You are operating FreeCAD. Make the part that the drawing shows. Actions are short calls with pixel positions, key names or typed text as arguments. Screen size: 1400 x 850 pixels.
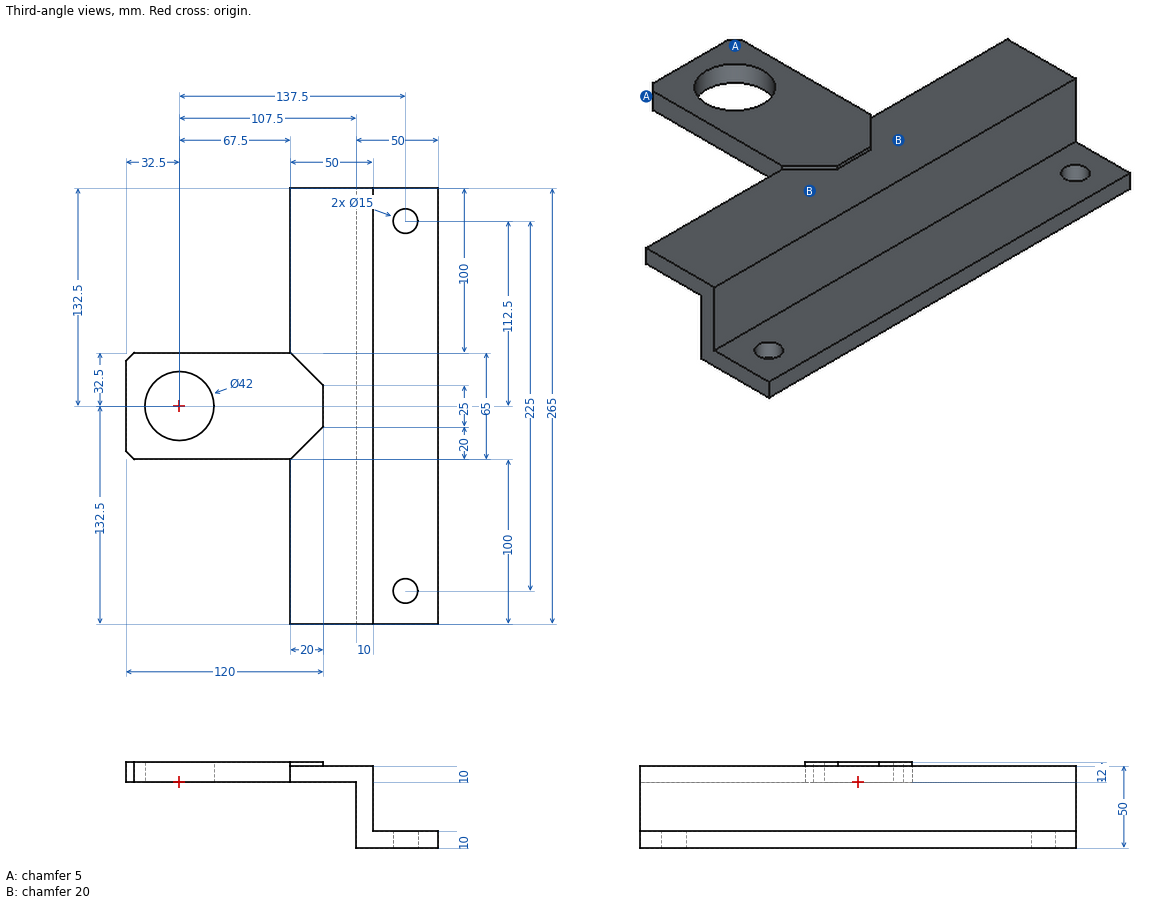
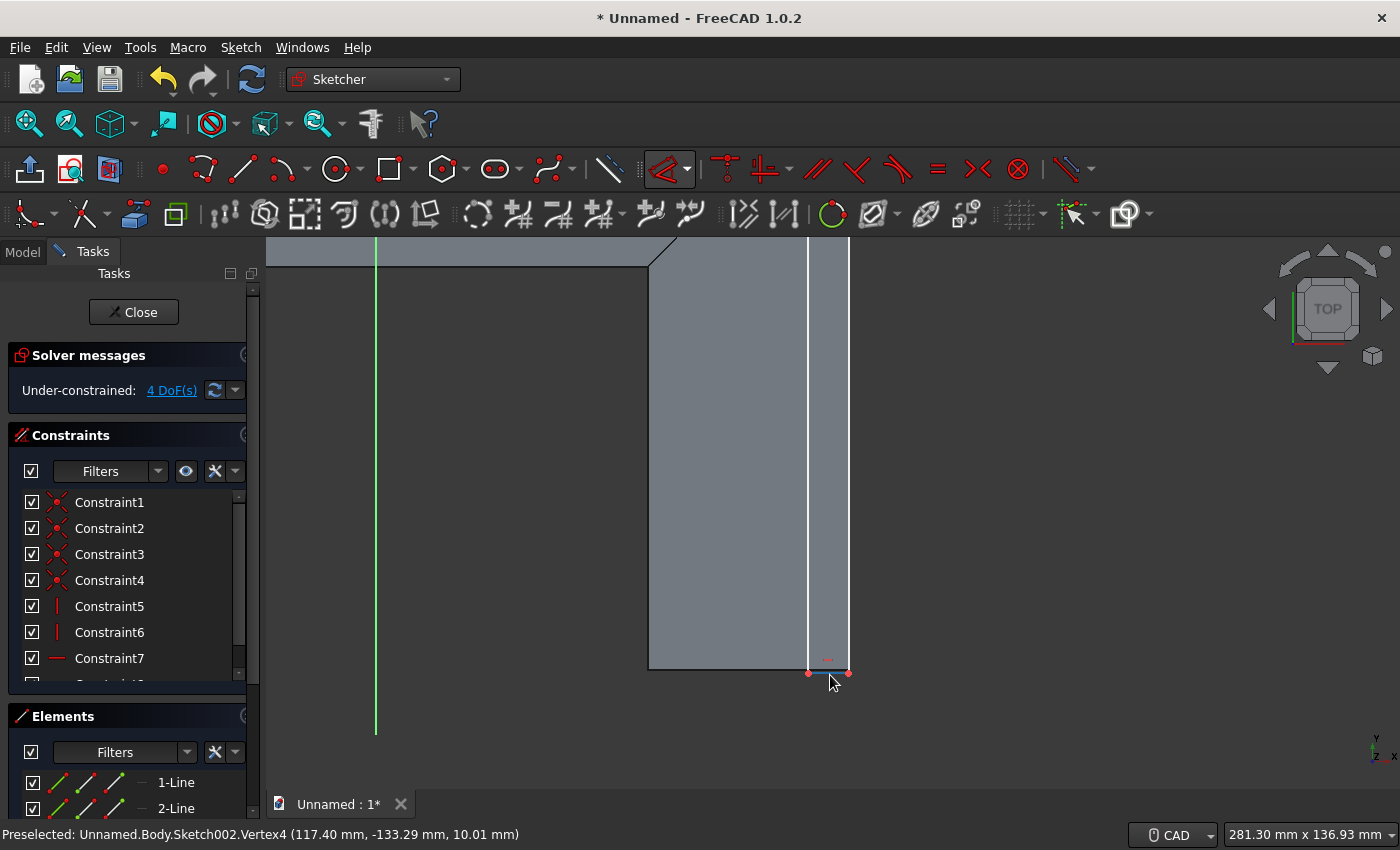
click(829, 673)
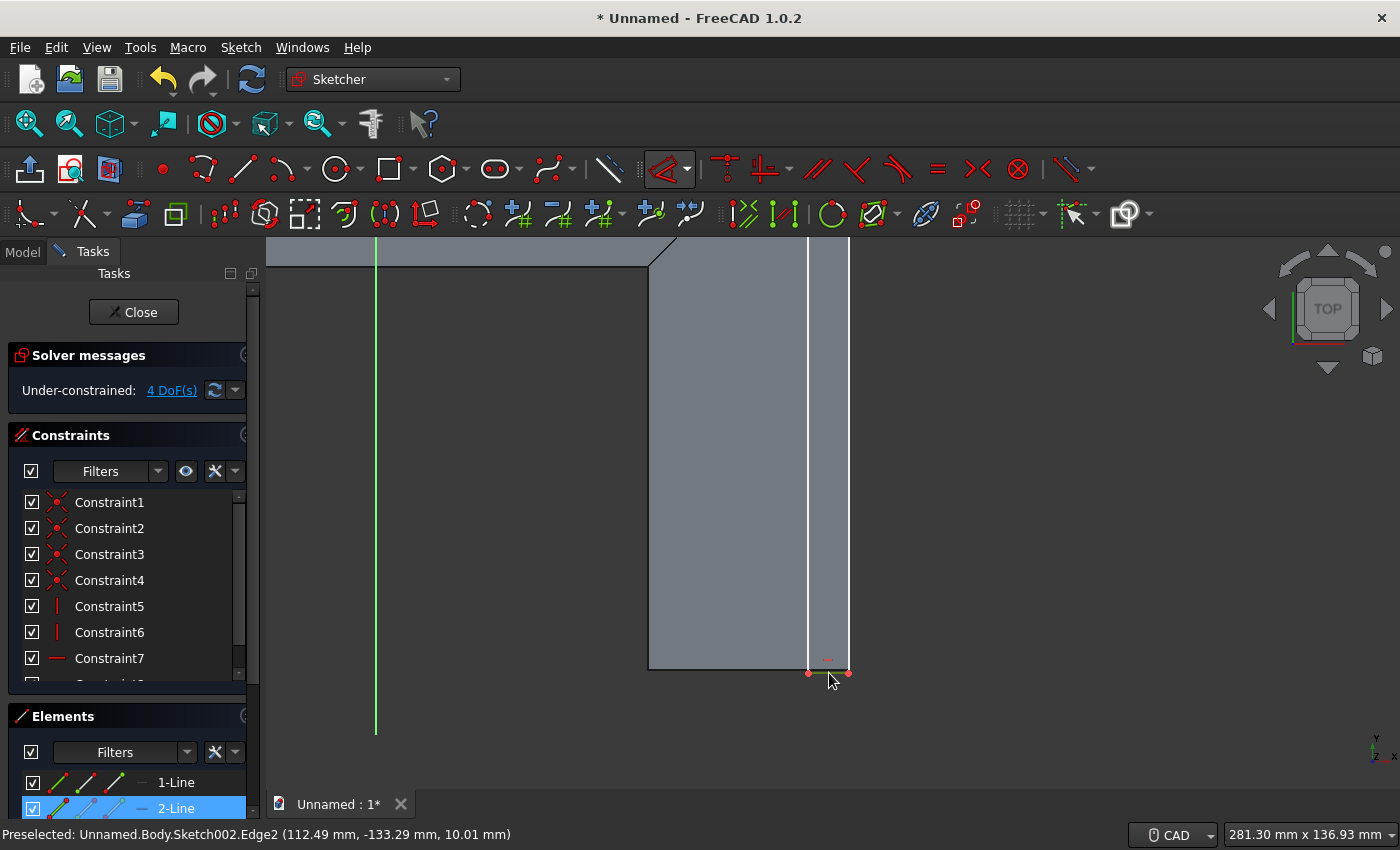
key(l)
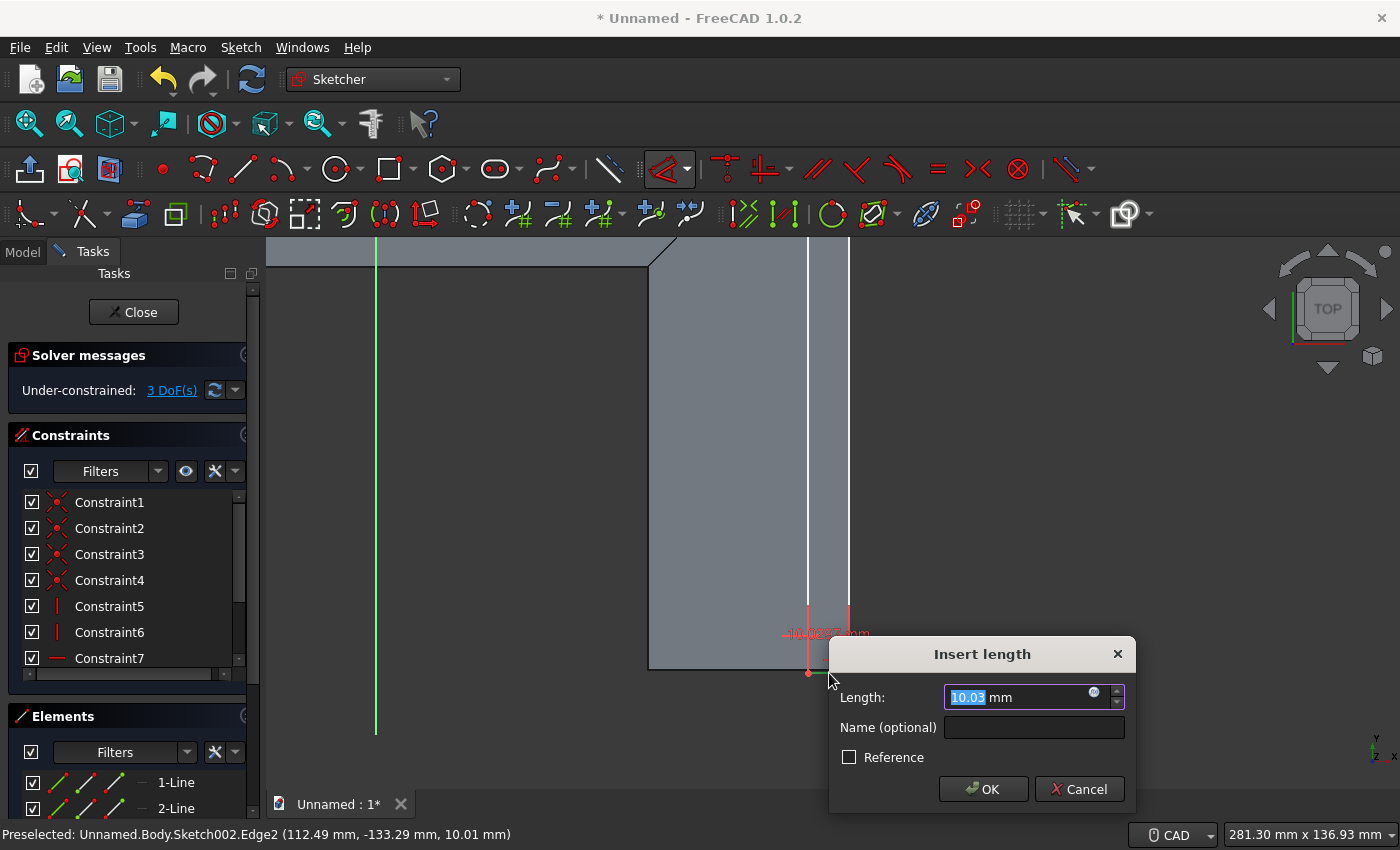
text(10)
key(Return)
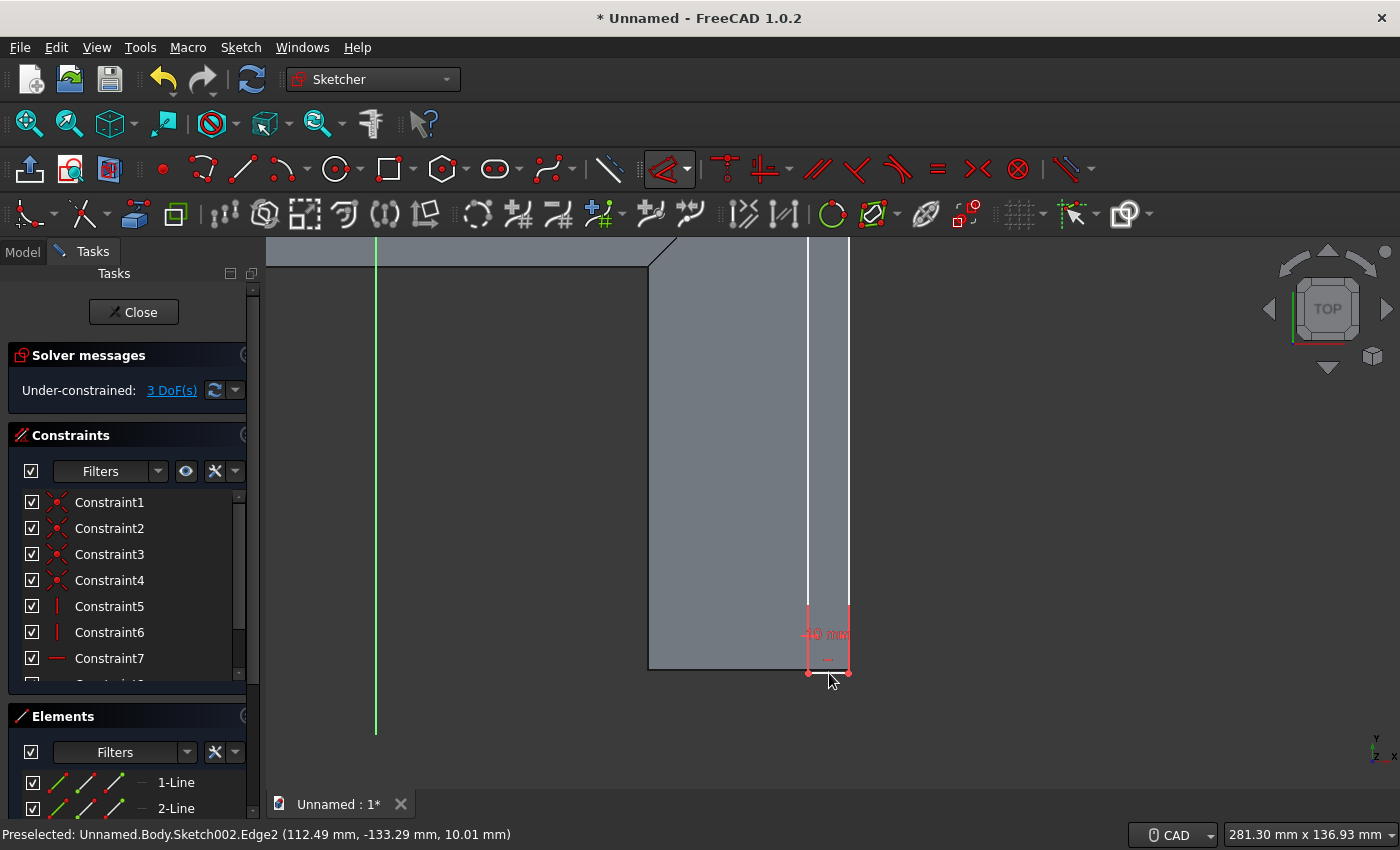
click(808, 352)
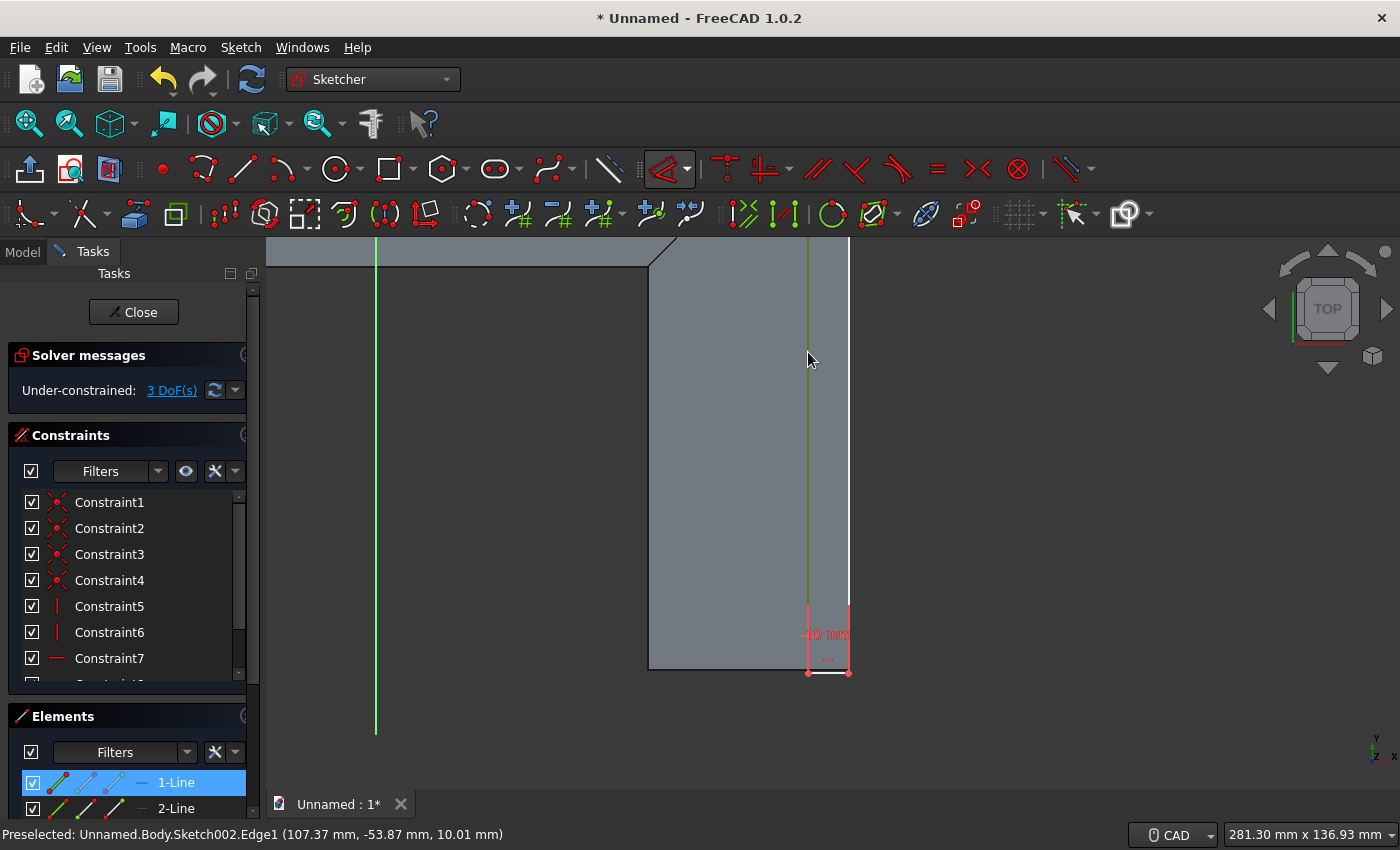
key(i)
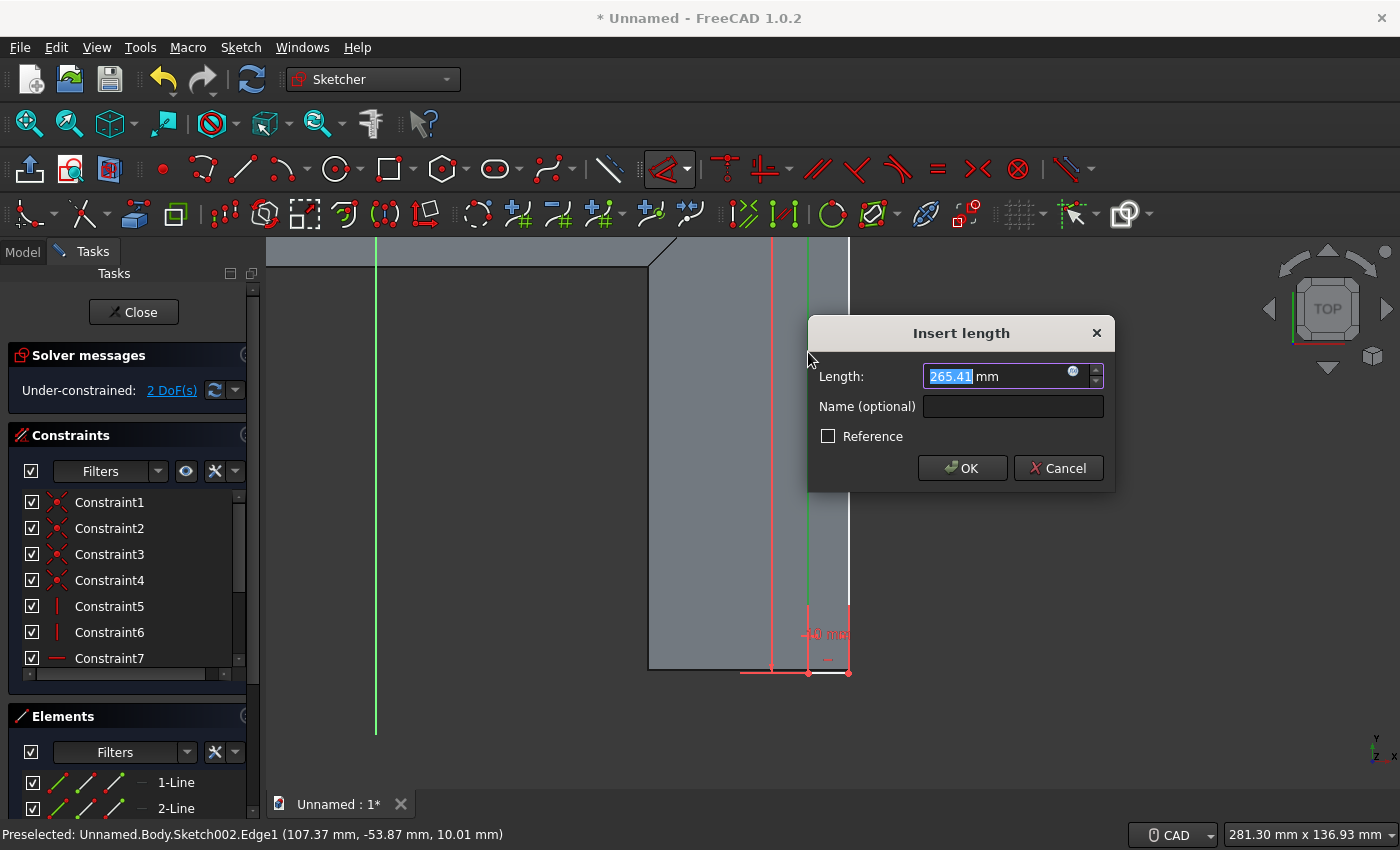
text(265)
key(Return)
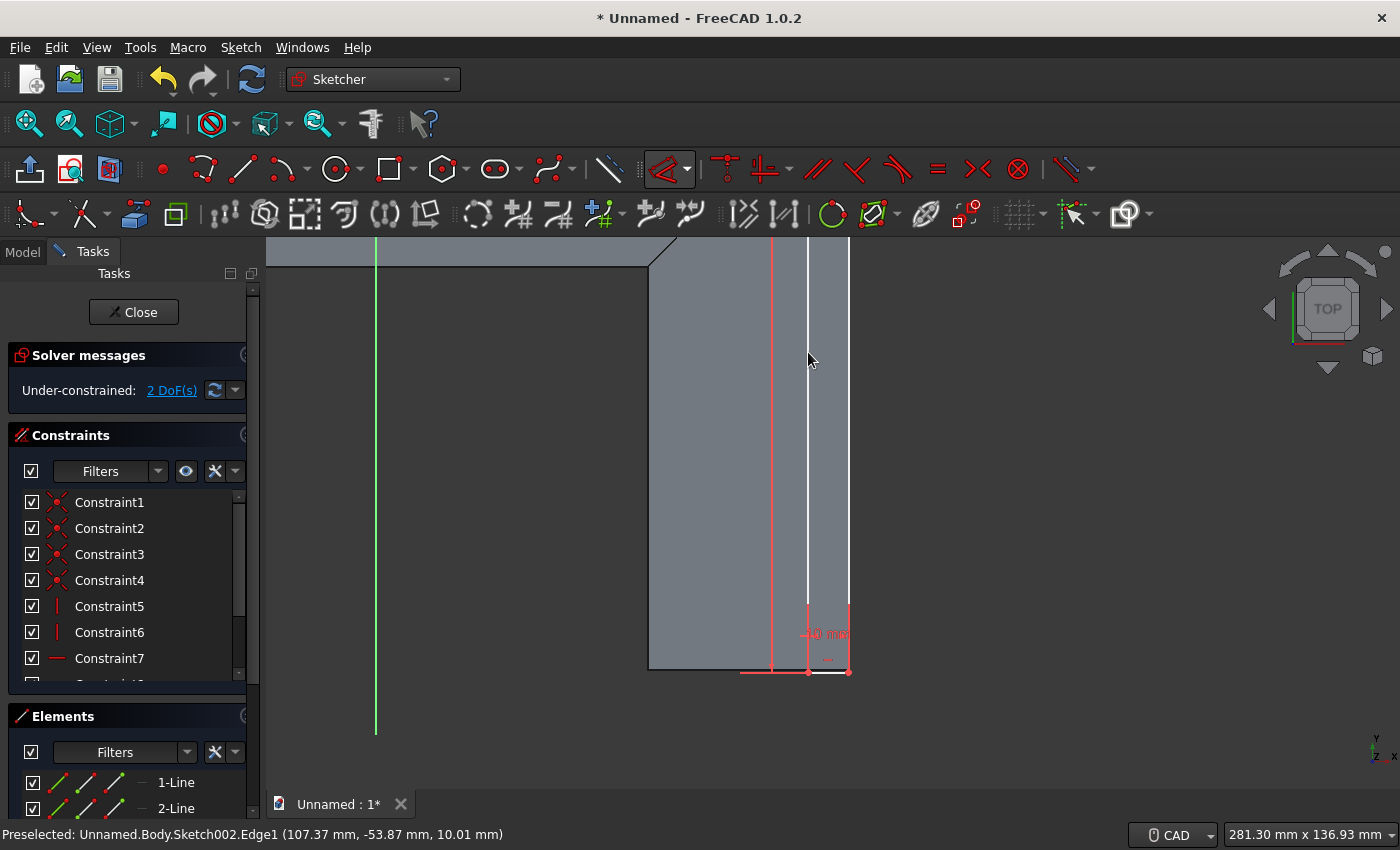
scroll(830, 676, down, 6)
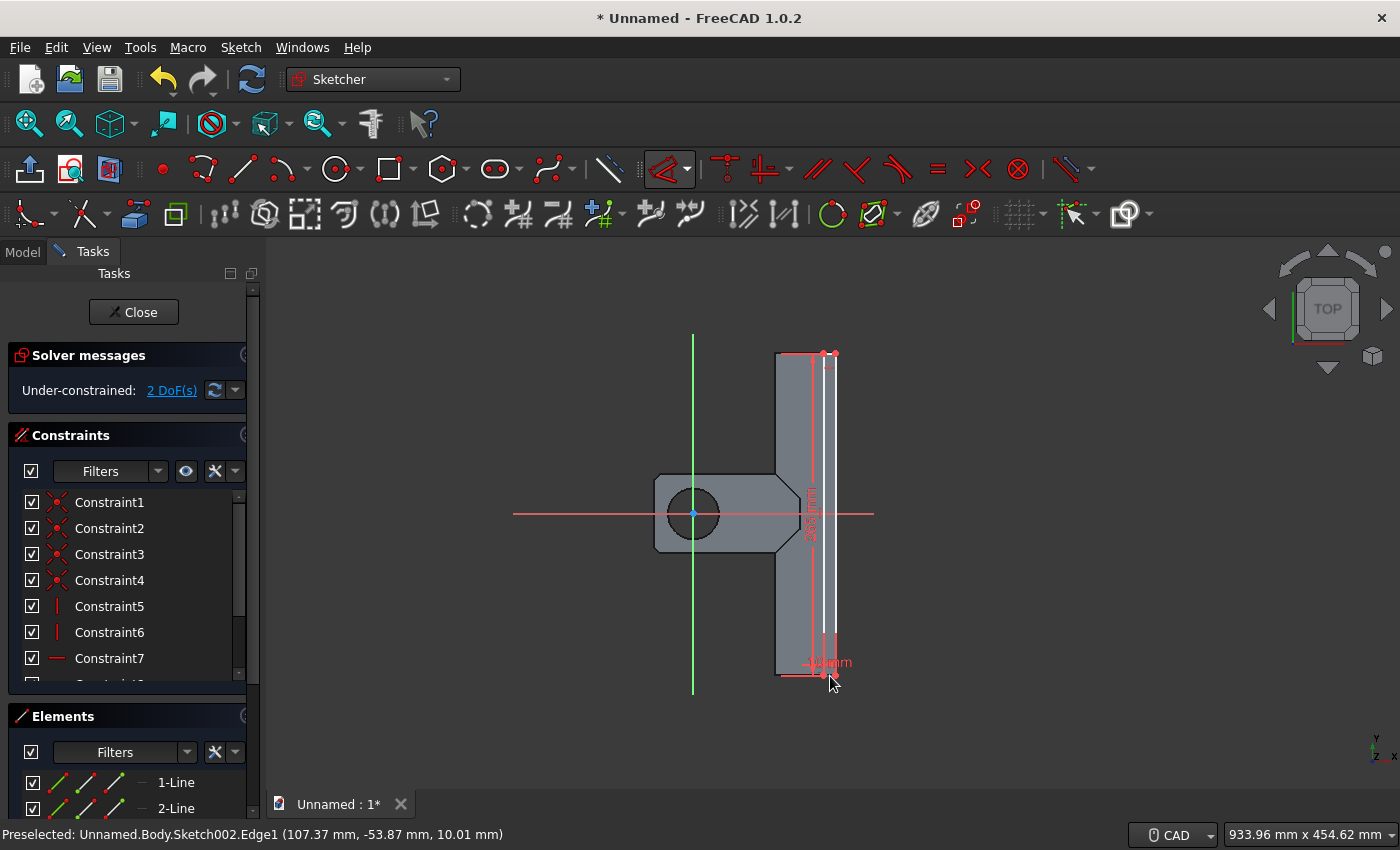
click(824, 354)